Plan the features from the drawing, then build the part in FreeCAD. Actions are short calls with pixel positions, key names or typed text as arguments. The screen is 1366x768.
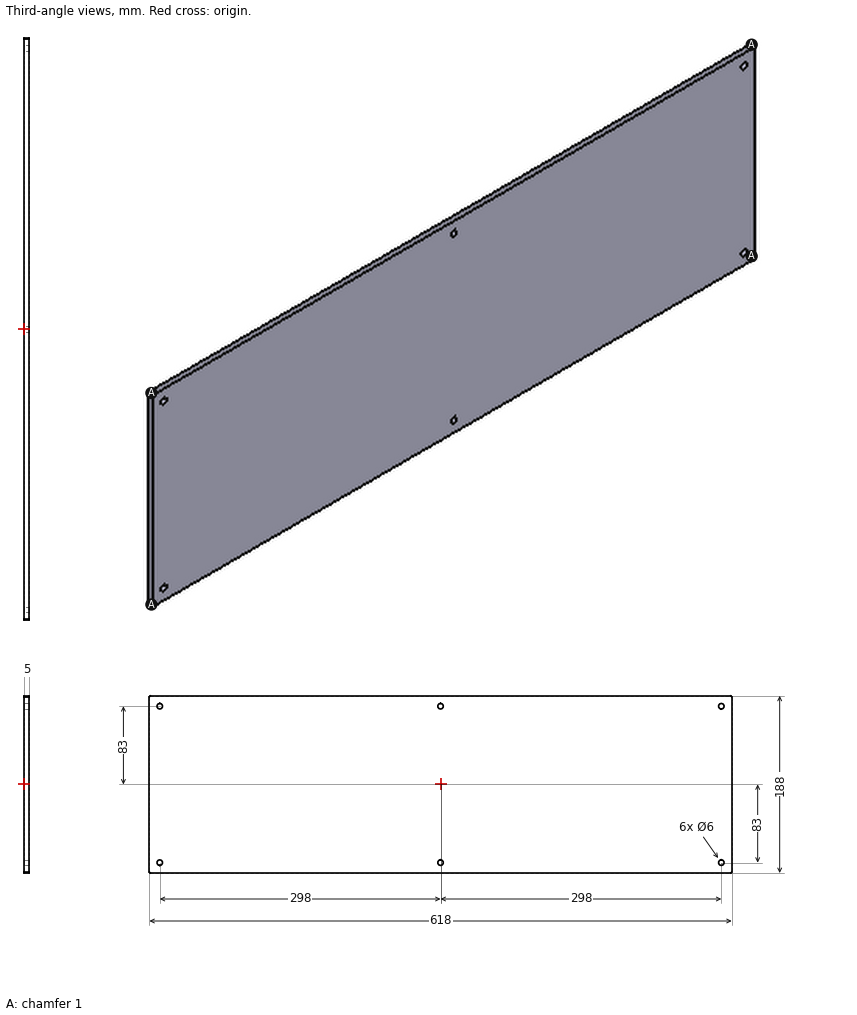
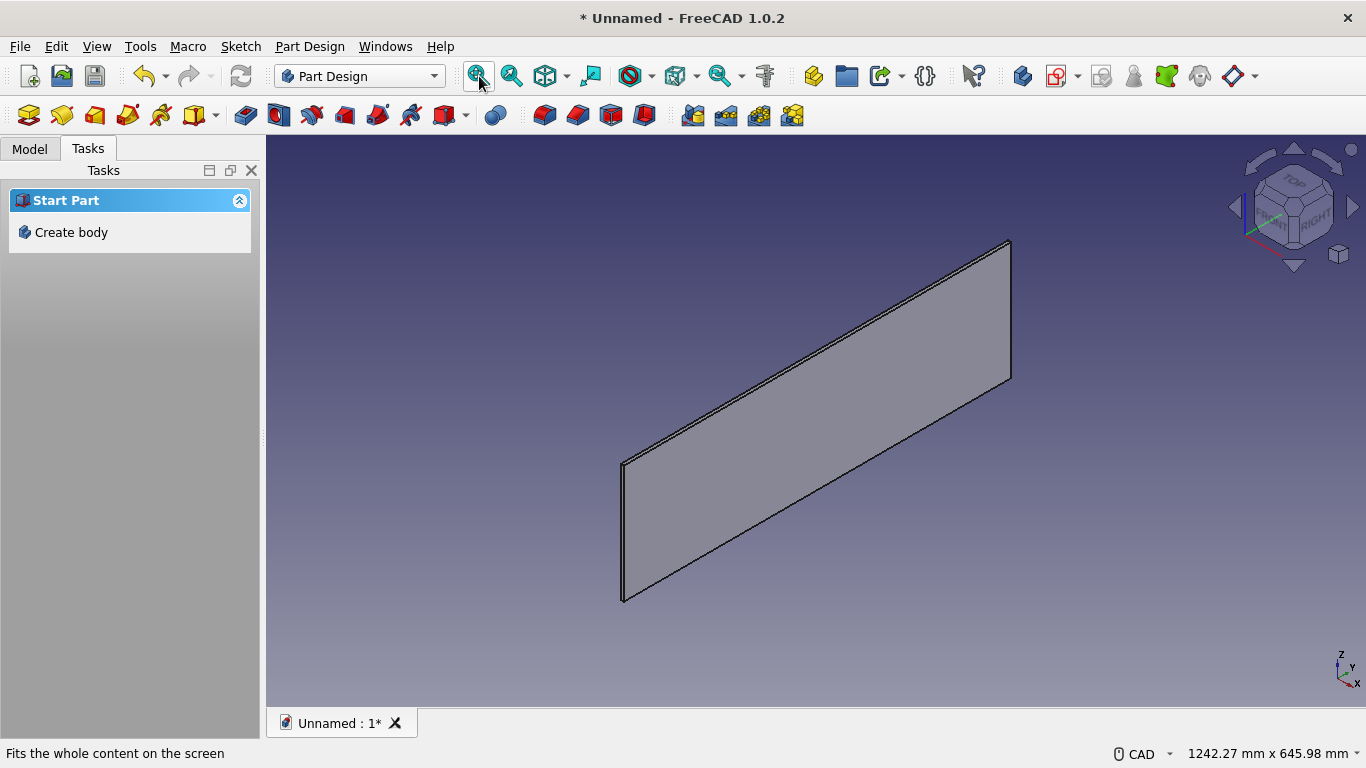
scroll(1009, 240, up, 12)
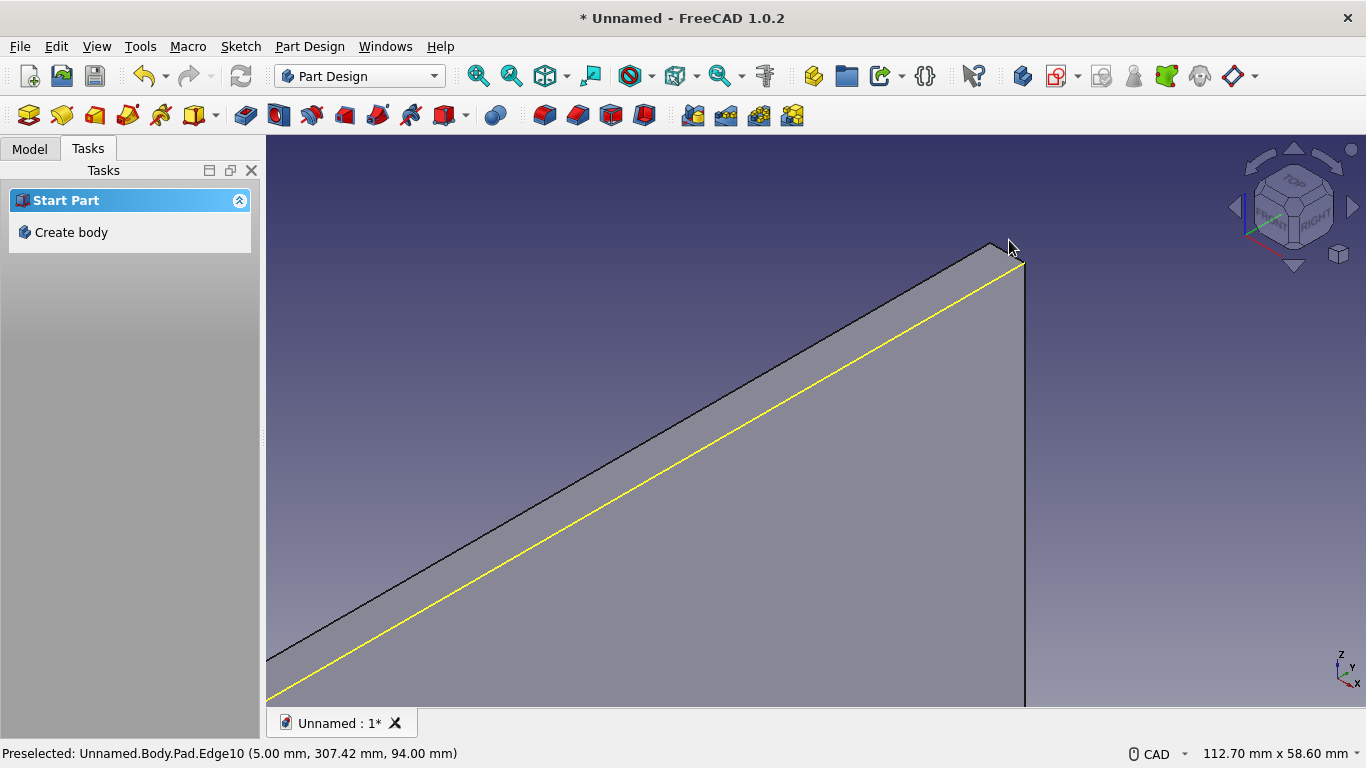
click(479, 76)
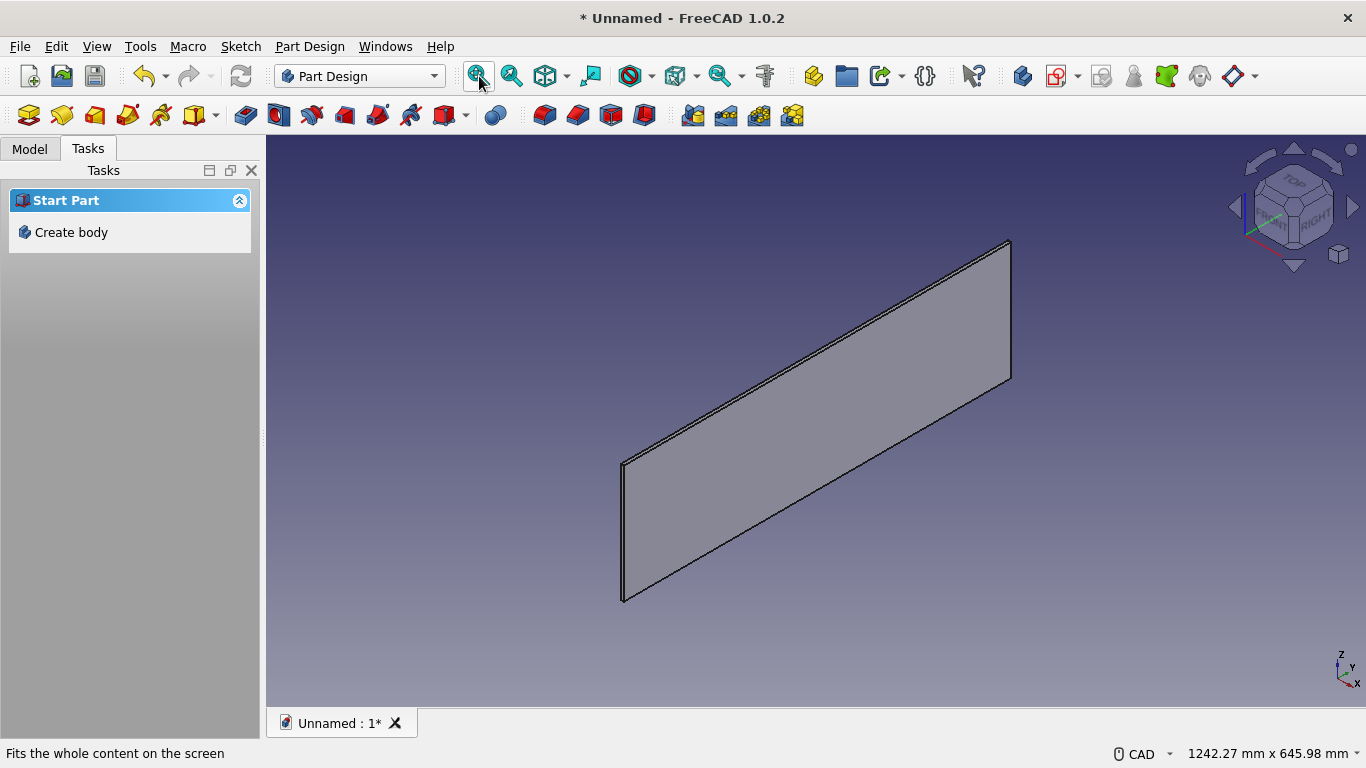
key(2)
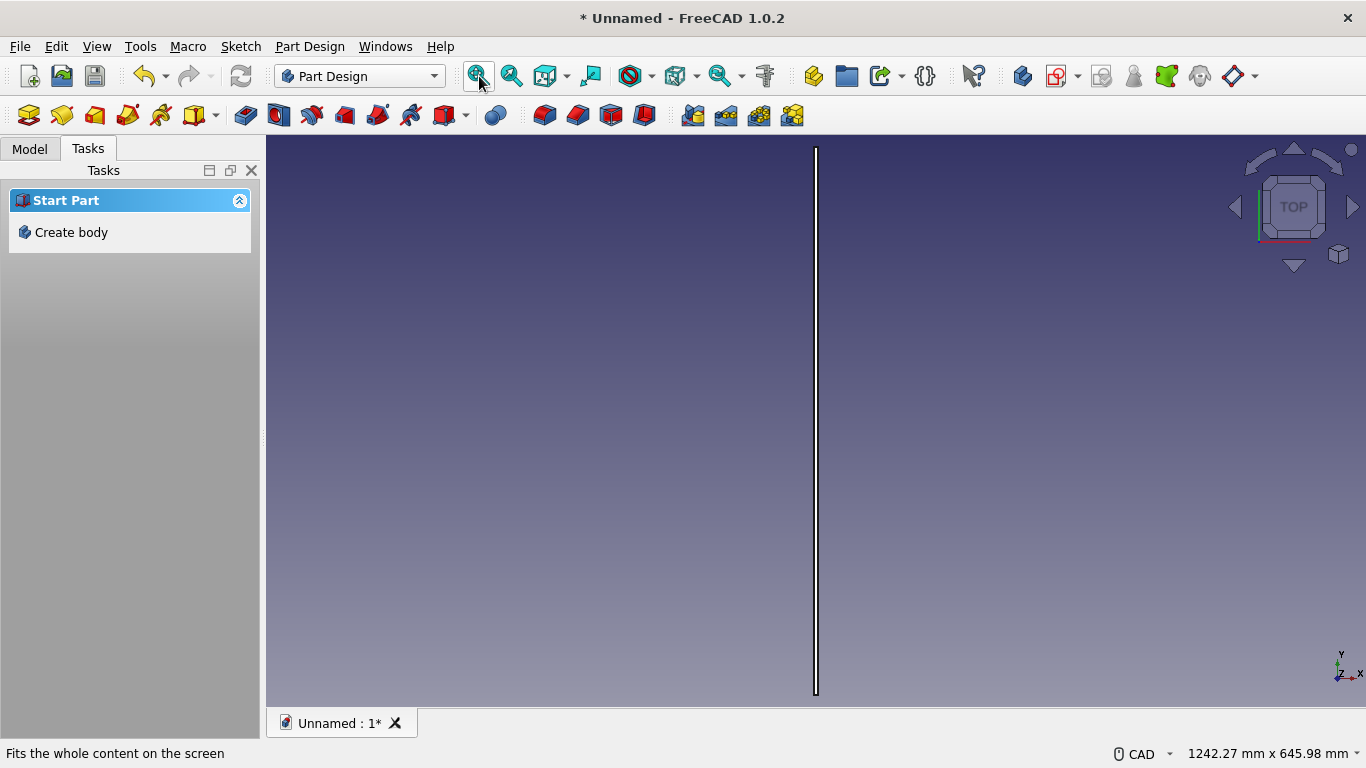
key(1)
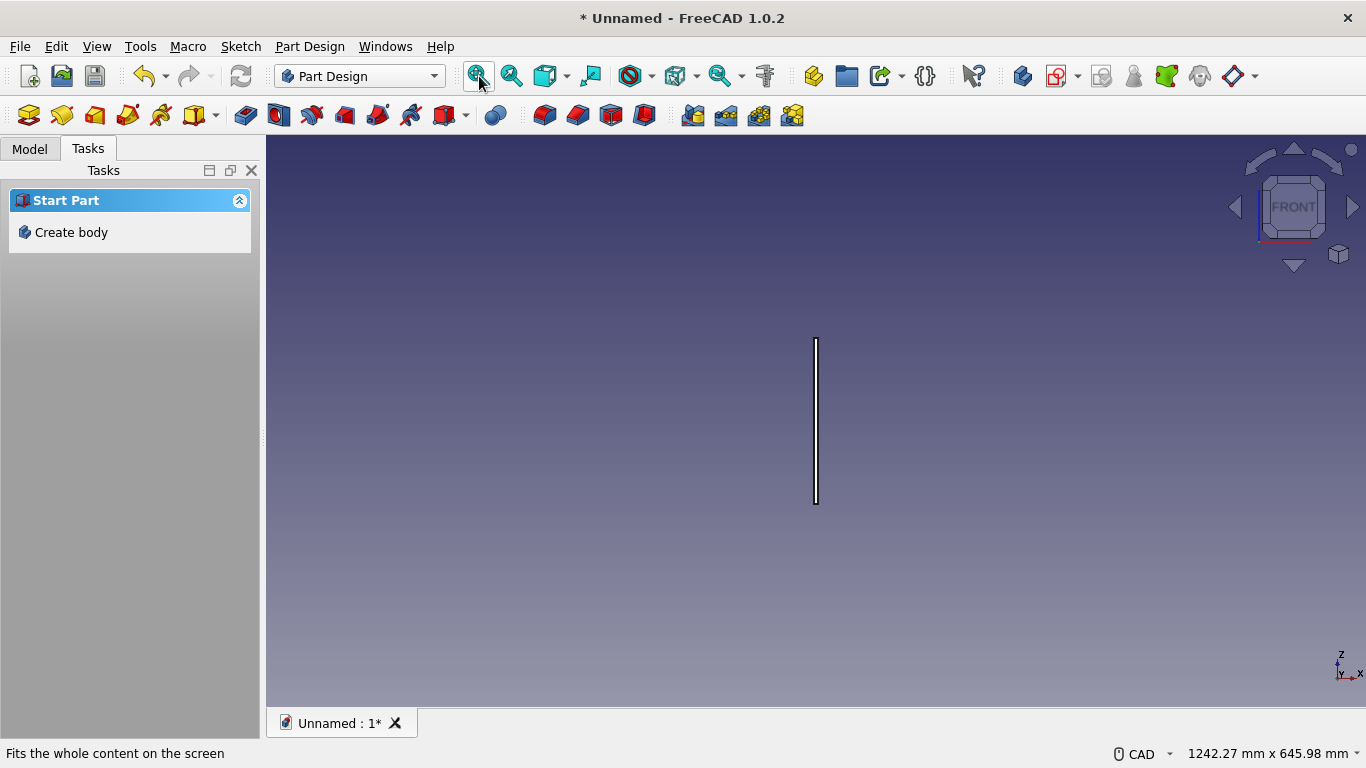
click(479, 76)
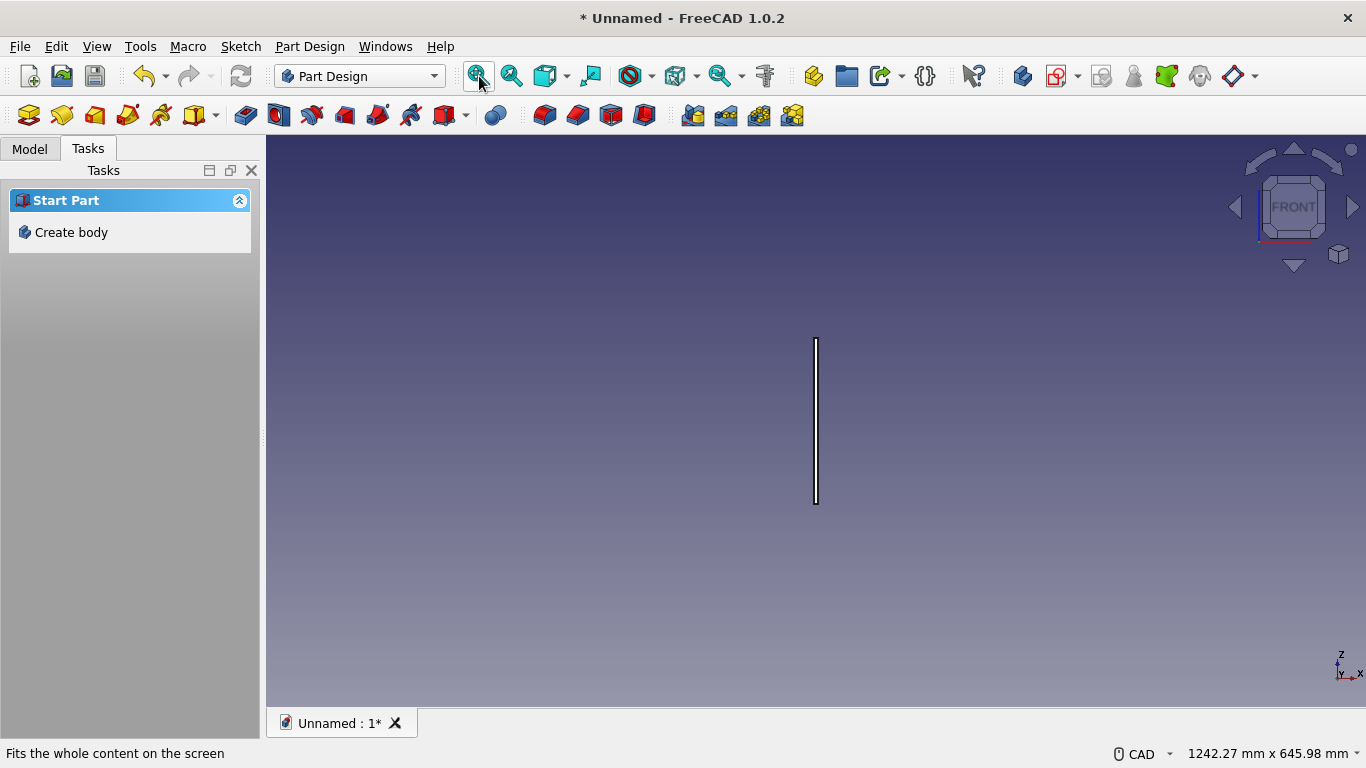
scroll(816, 337, up, 12)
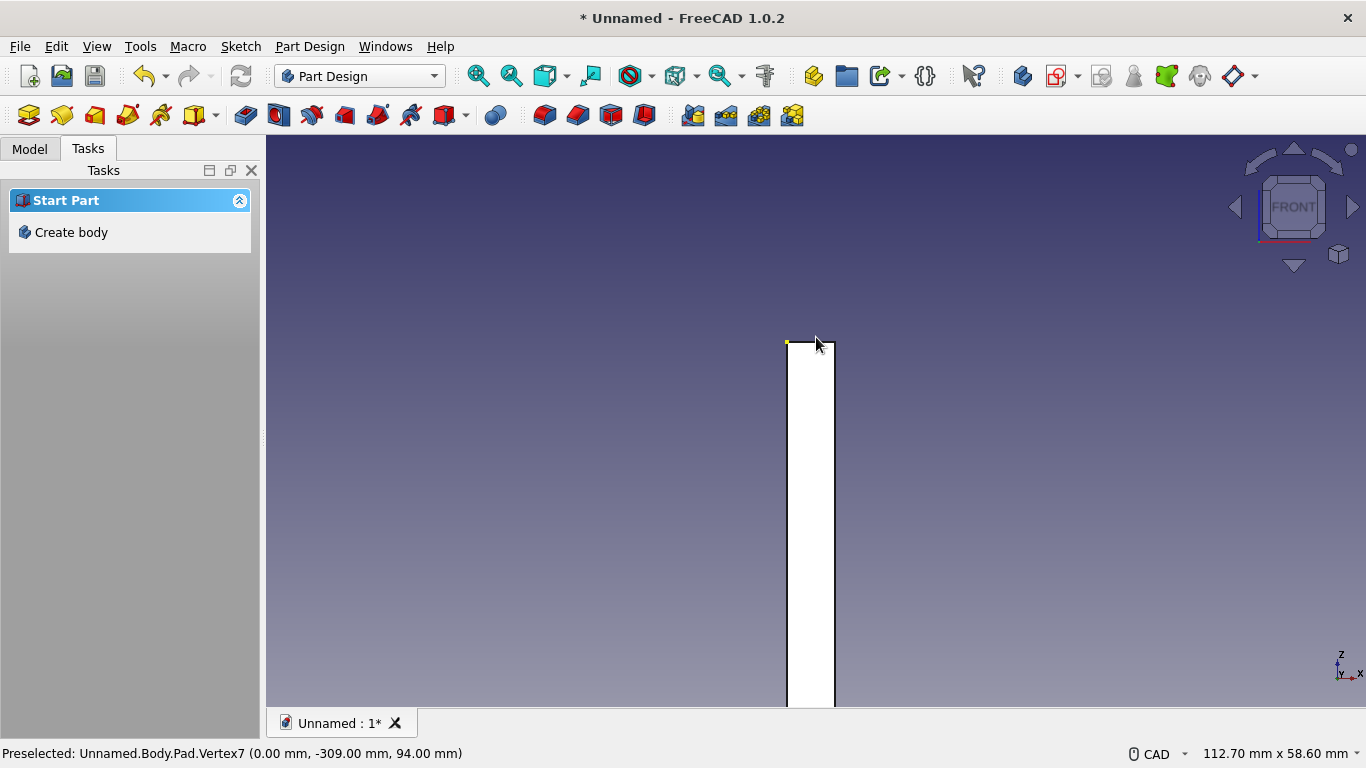
click(811, 341)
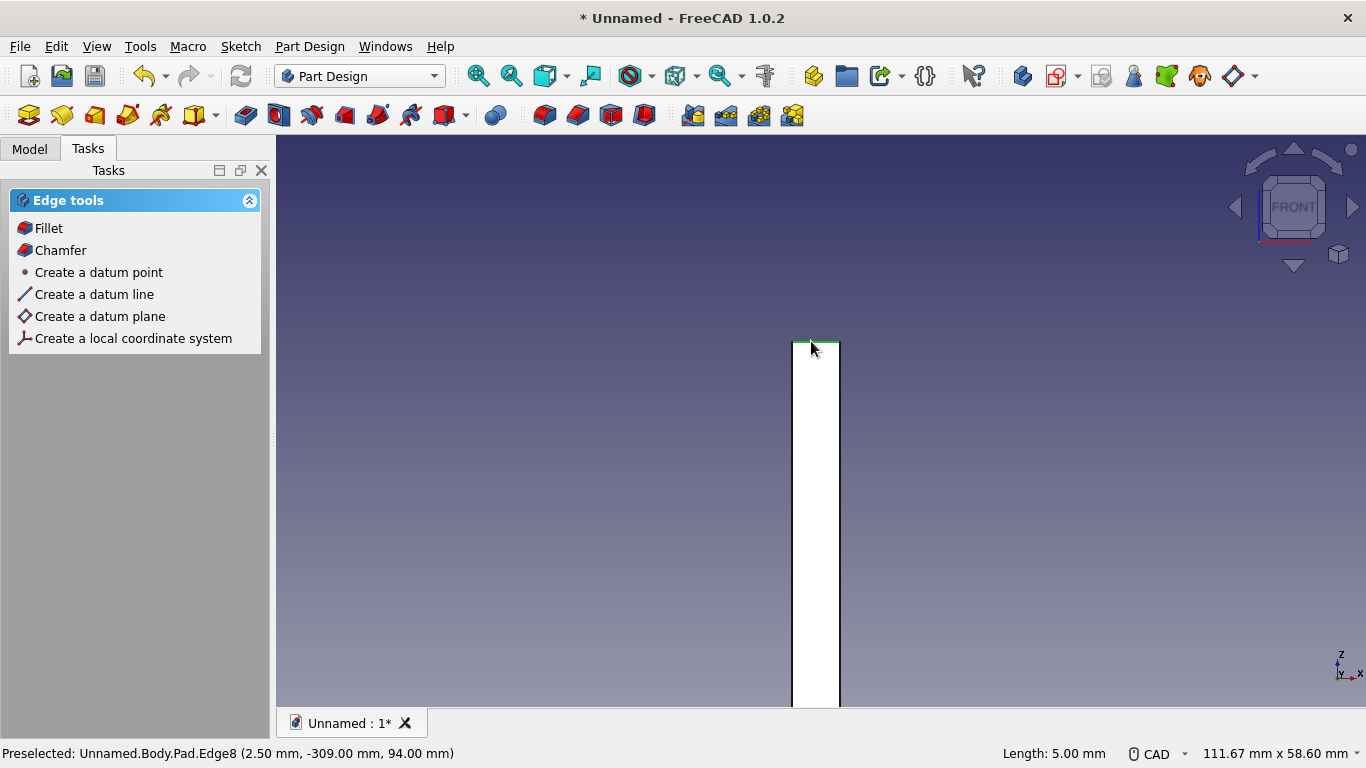
click(479, 76)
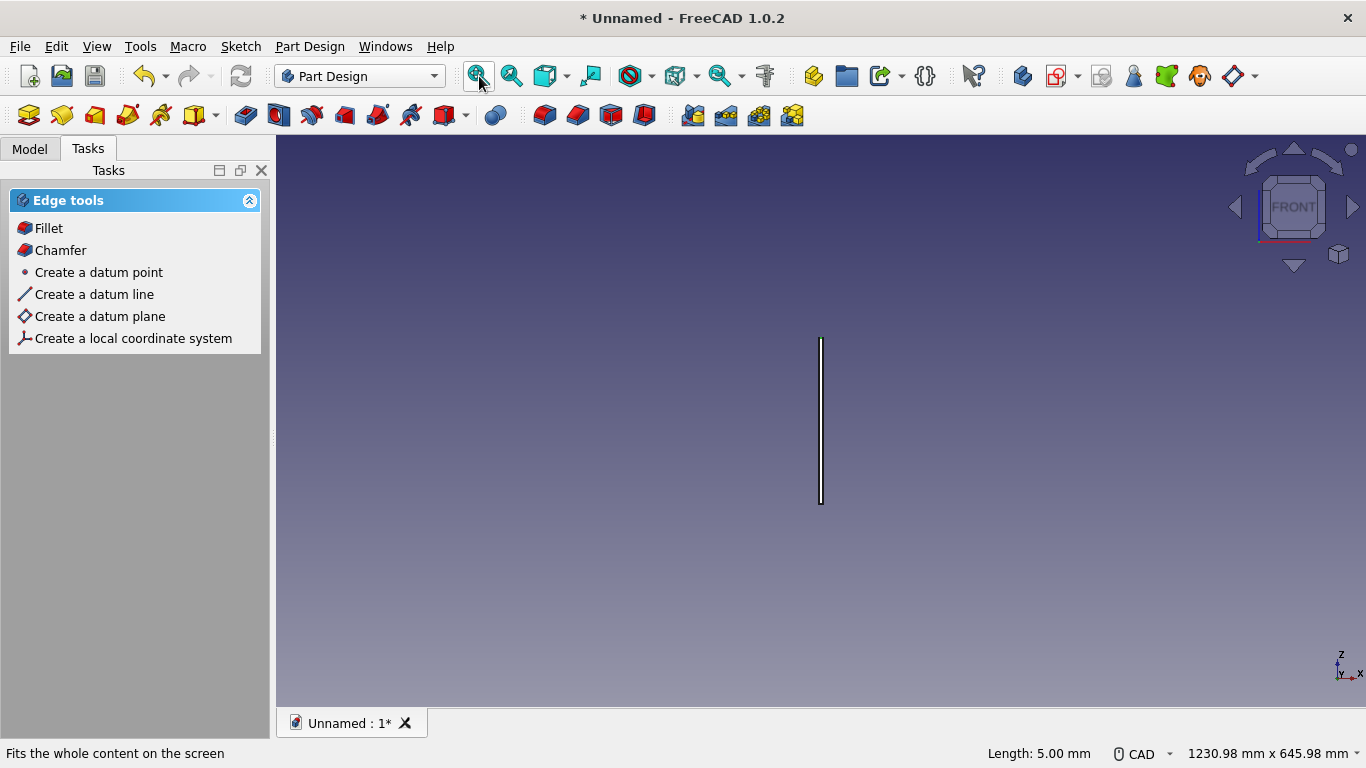
key(3)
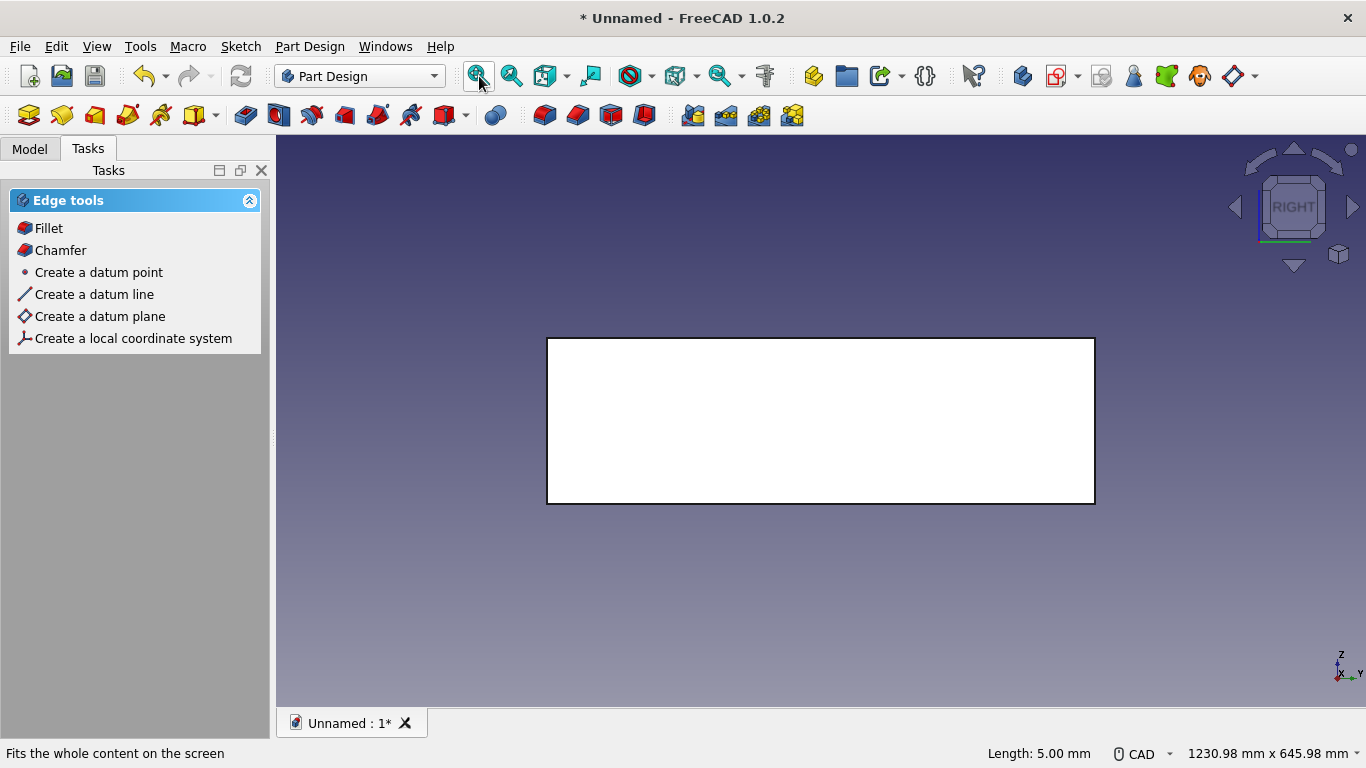
scroll(1095, 337, up, 12)